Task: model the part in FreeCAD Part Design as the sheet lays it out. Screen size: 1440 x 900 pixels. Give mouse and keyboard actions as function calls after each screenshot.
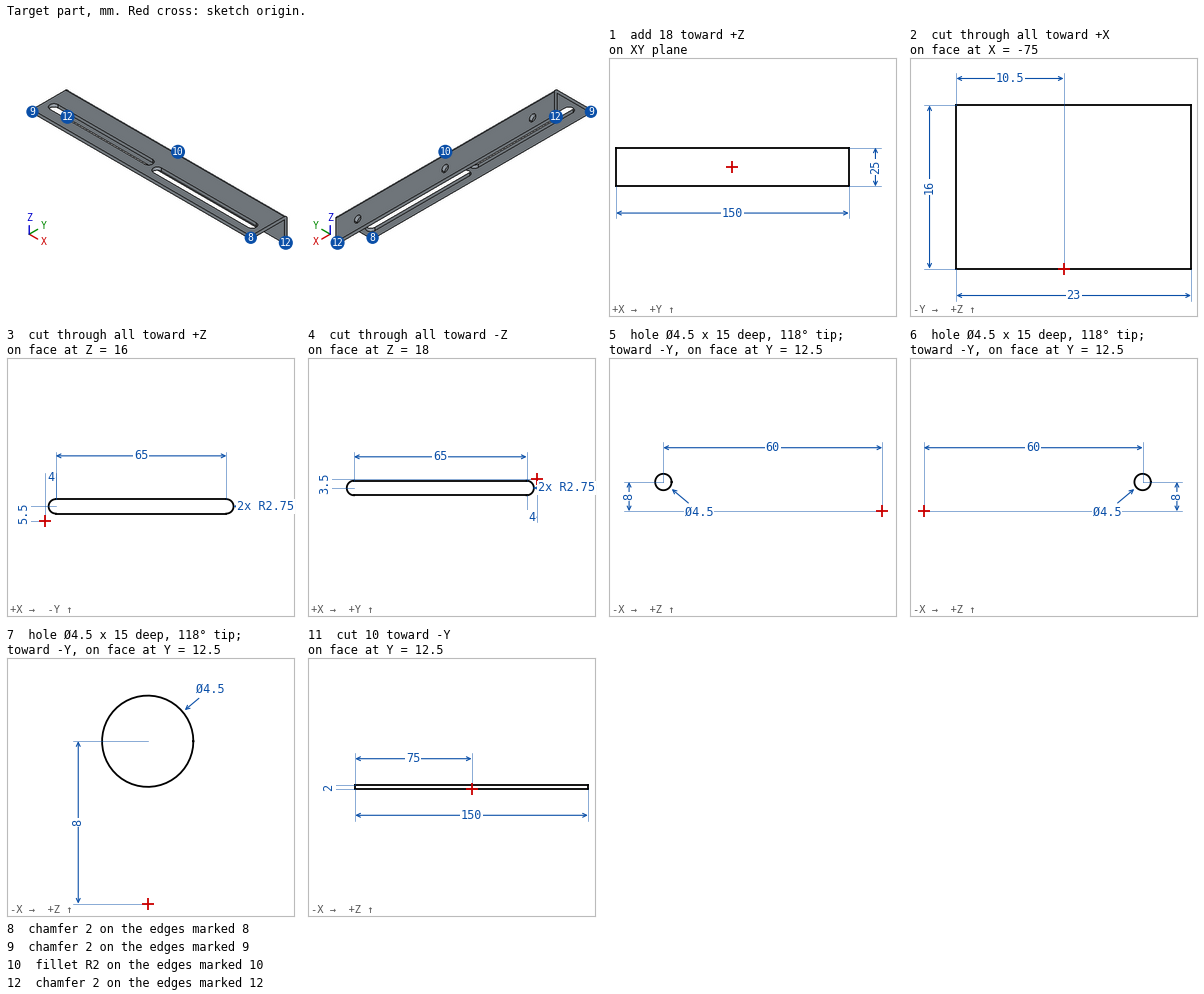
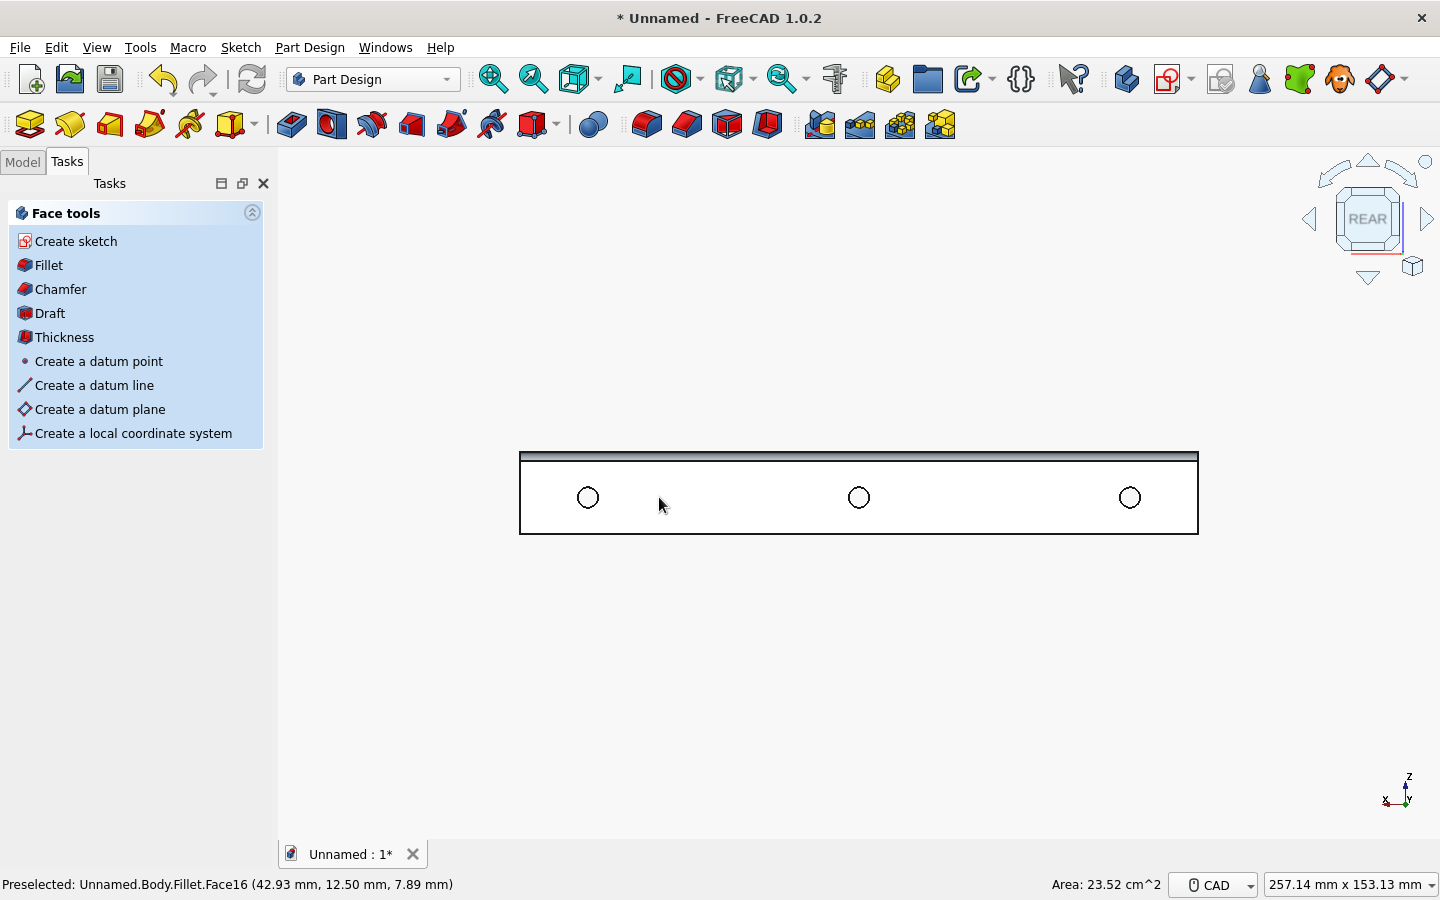
click(1168, 80)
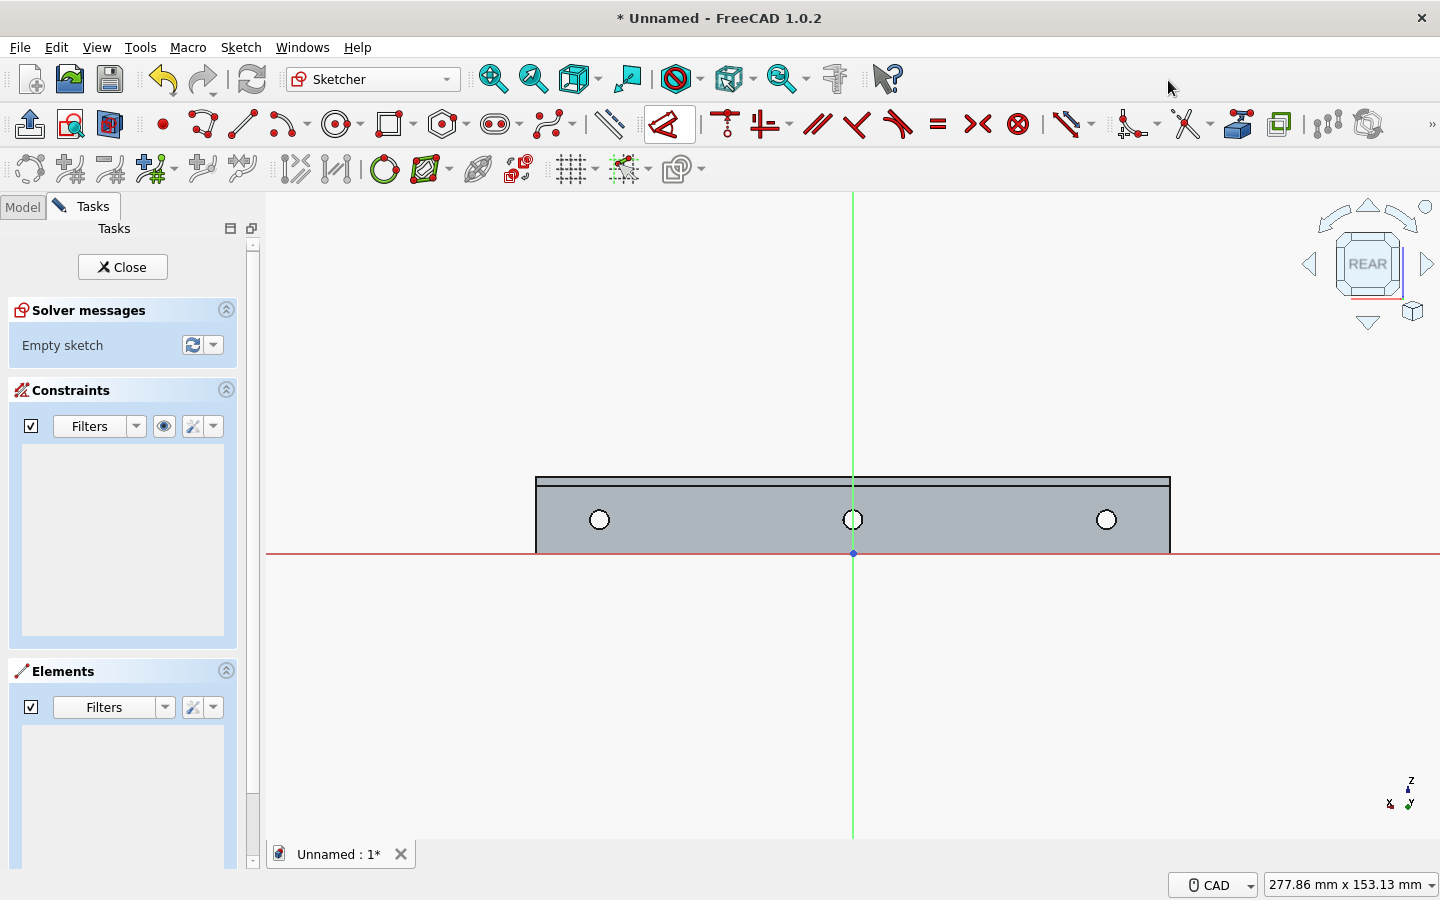
click(390, 124)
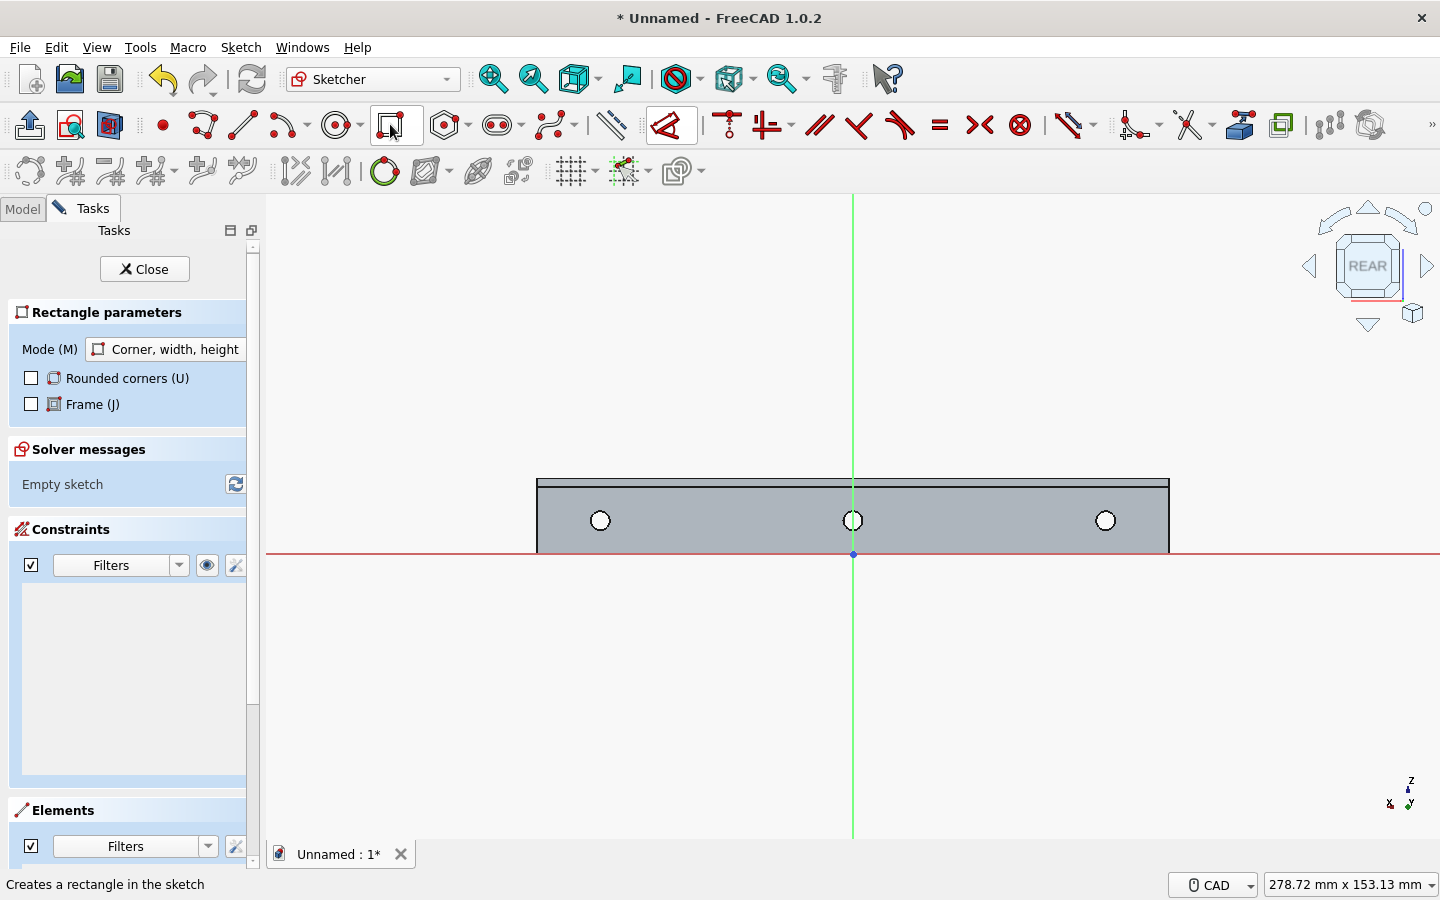
scroll(537, 546, up, 4)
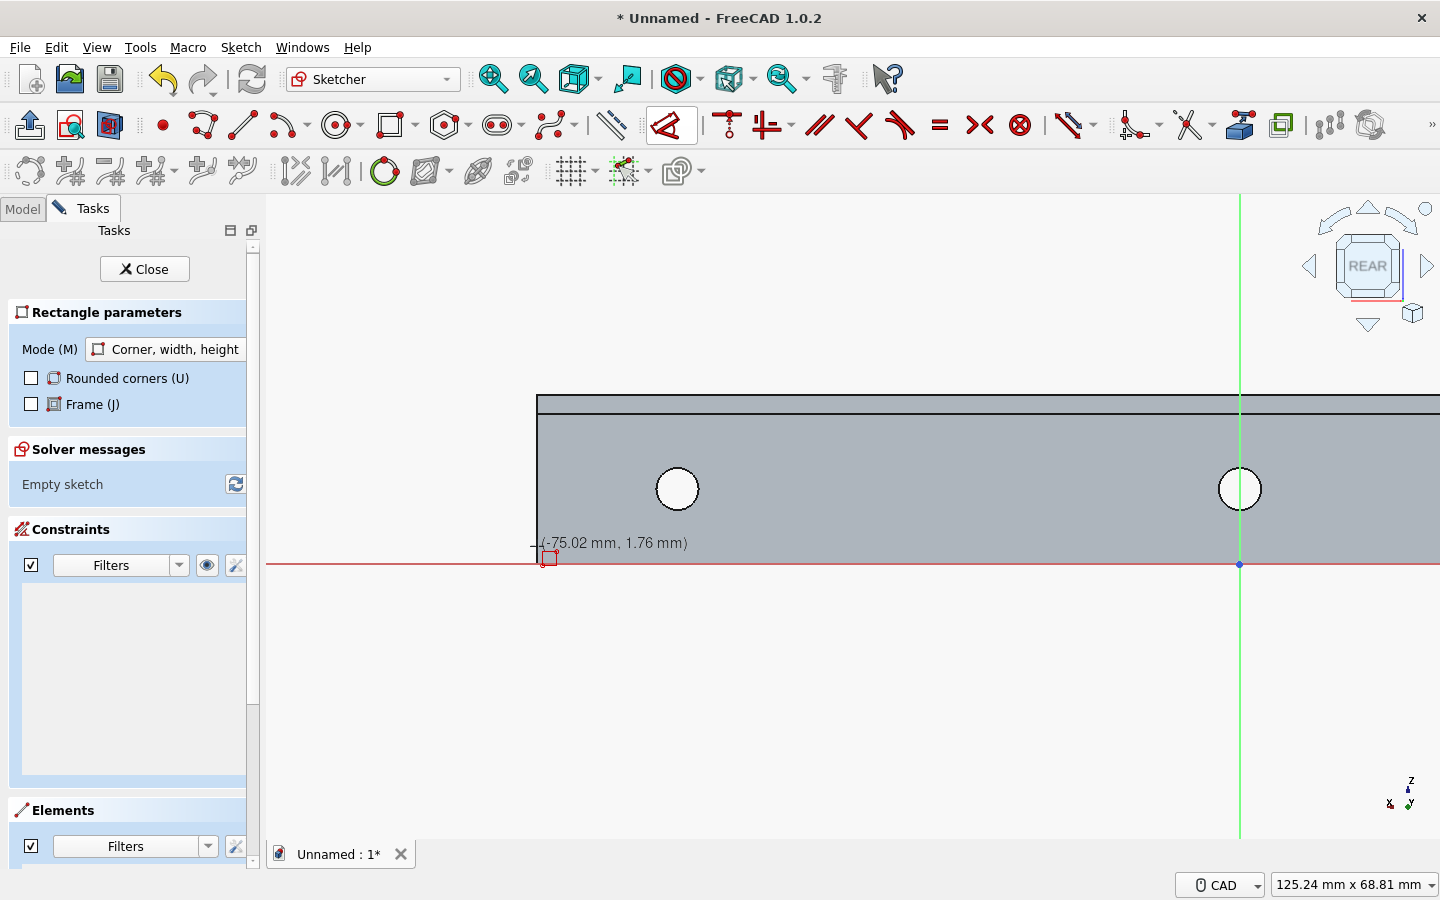
click(537, 545)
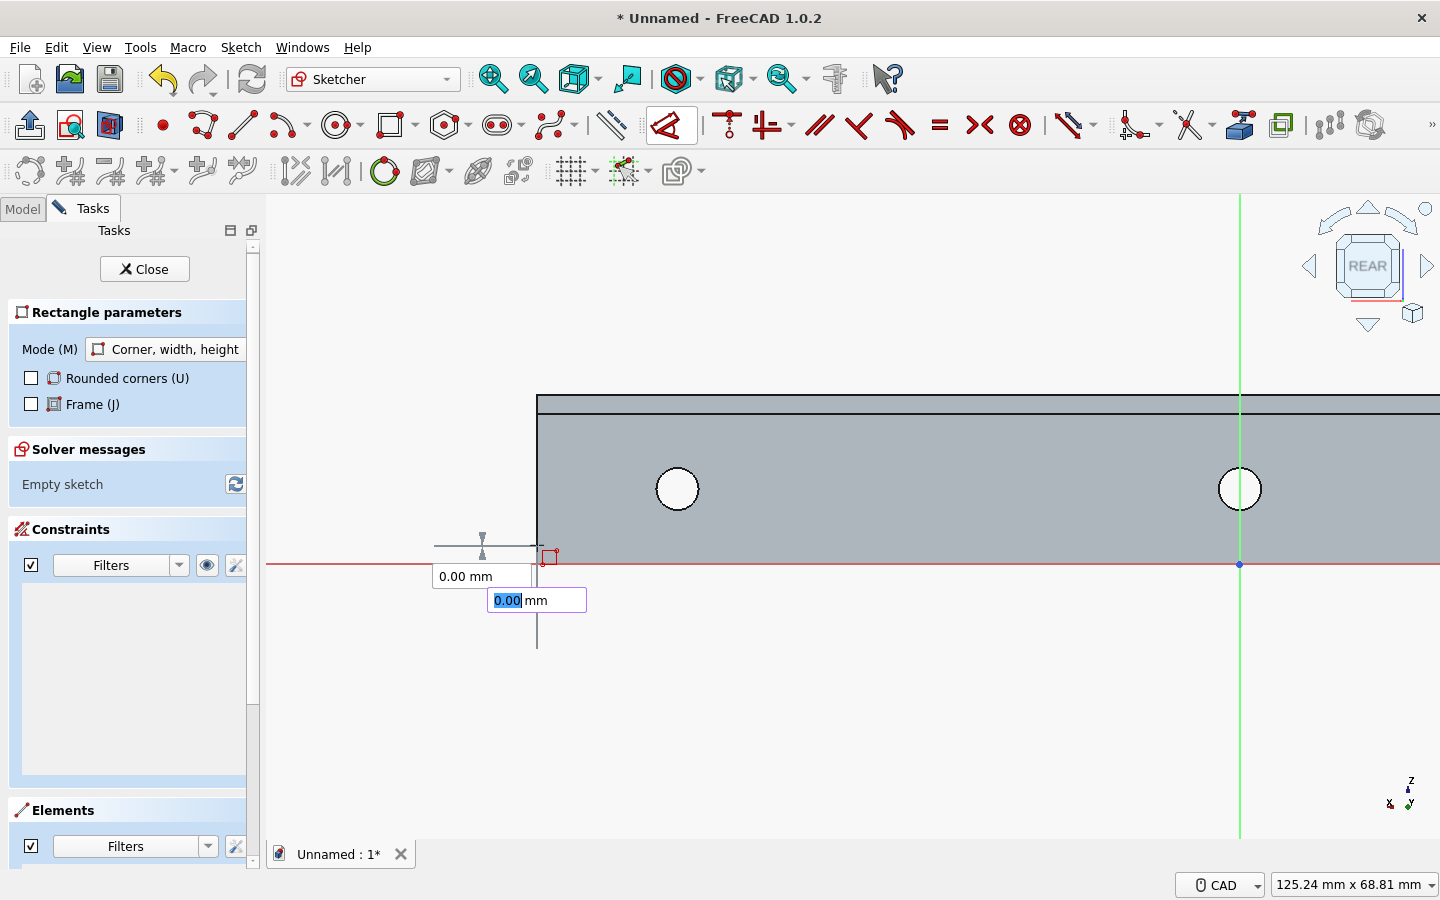
scroll(413, 485, down, 4)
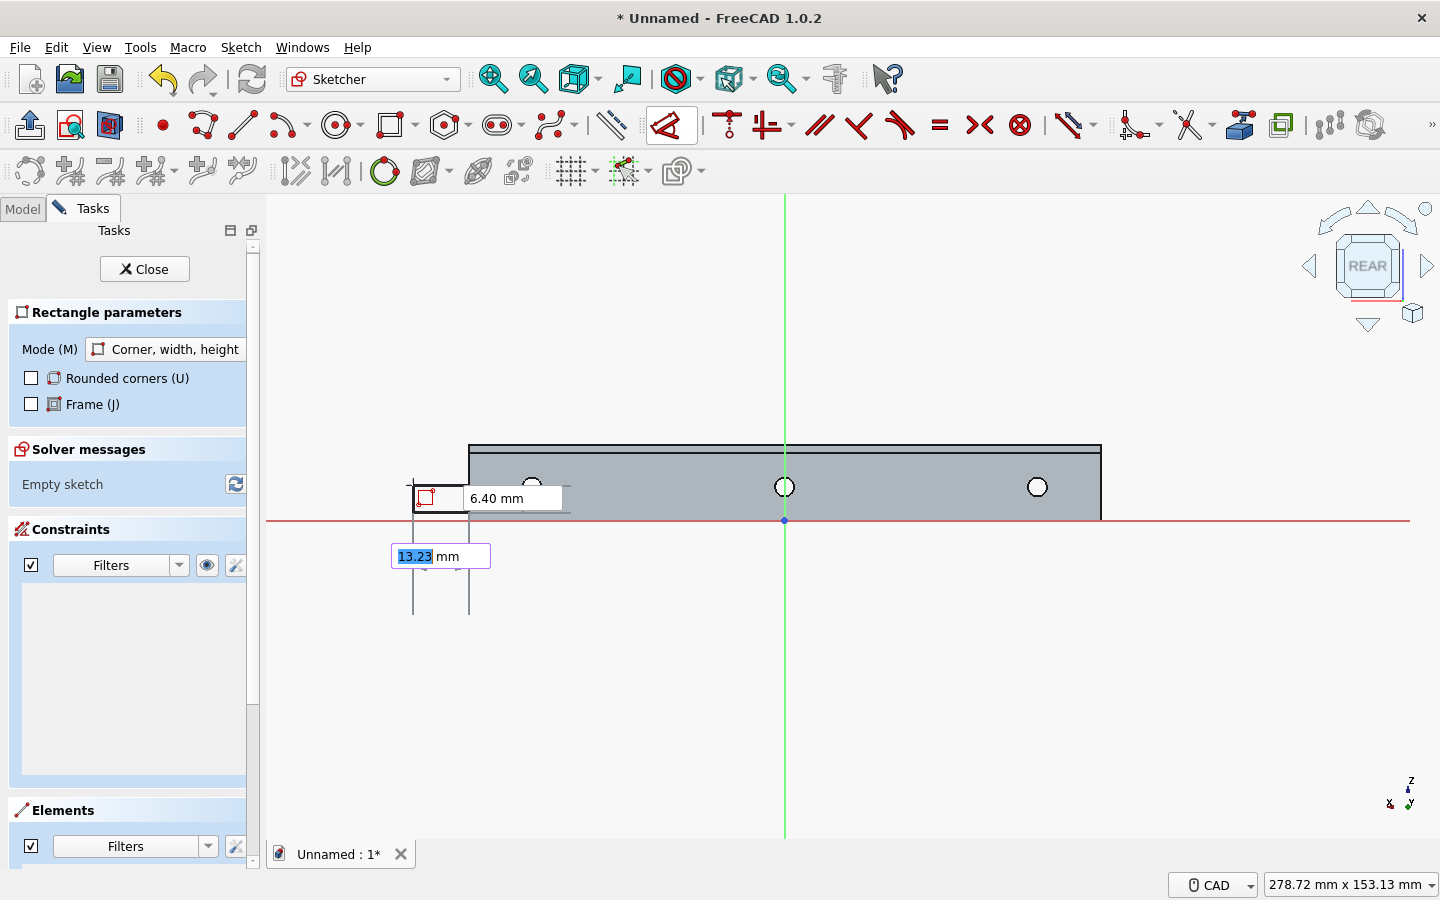
click(1101, 521)
key(Escape)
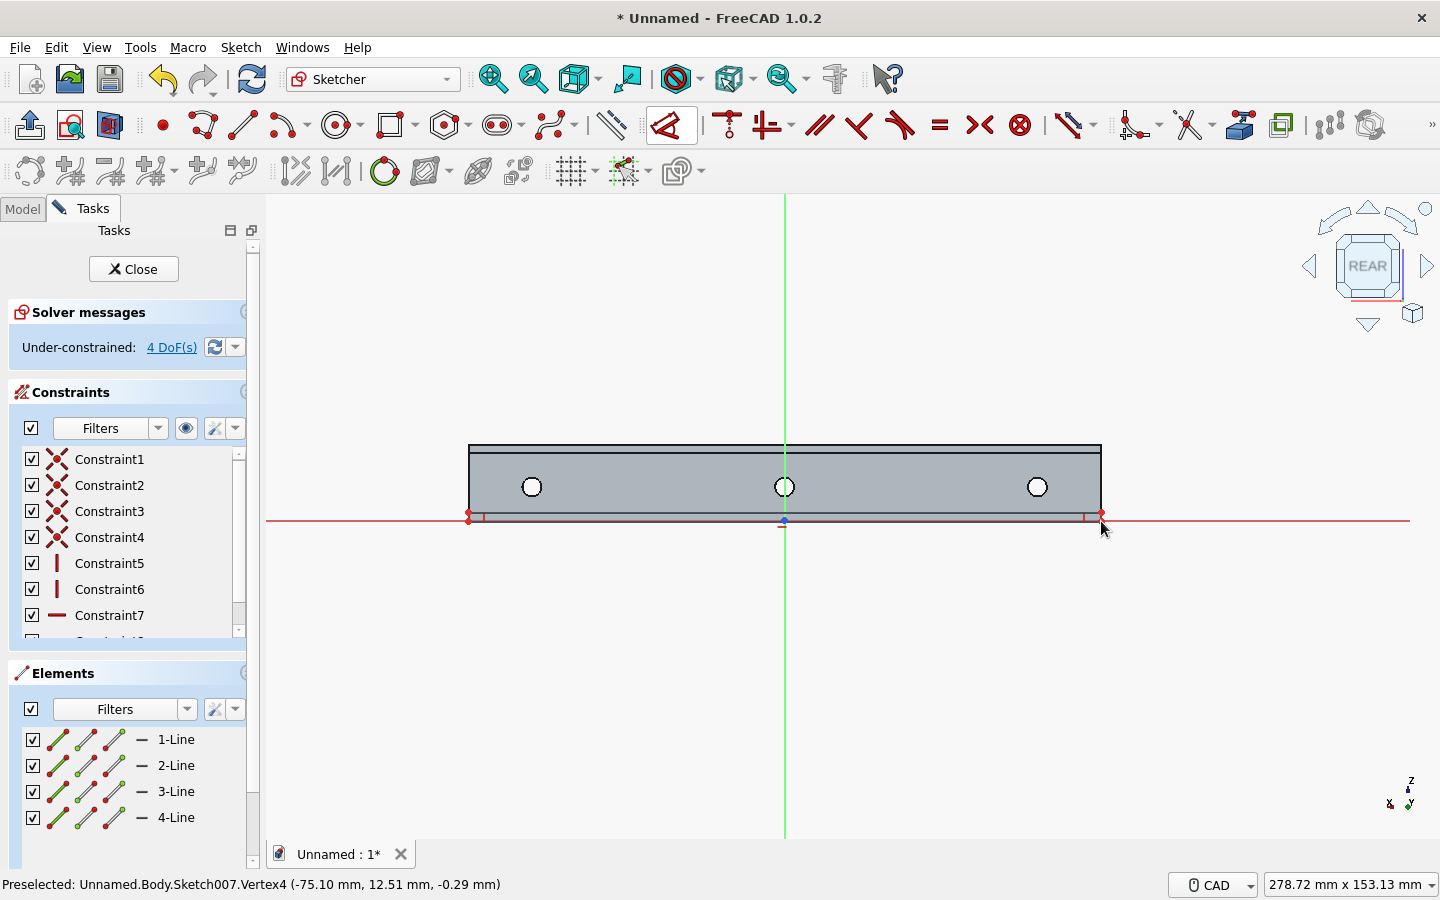
scroll(469, 522, up, 2)